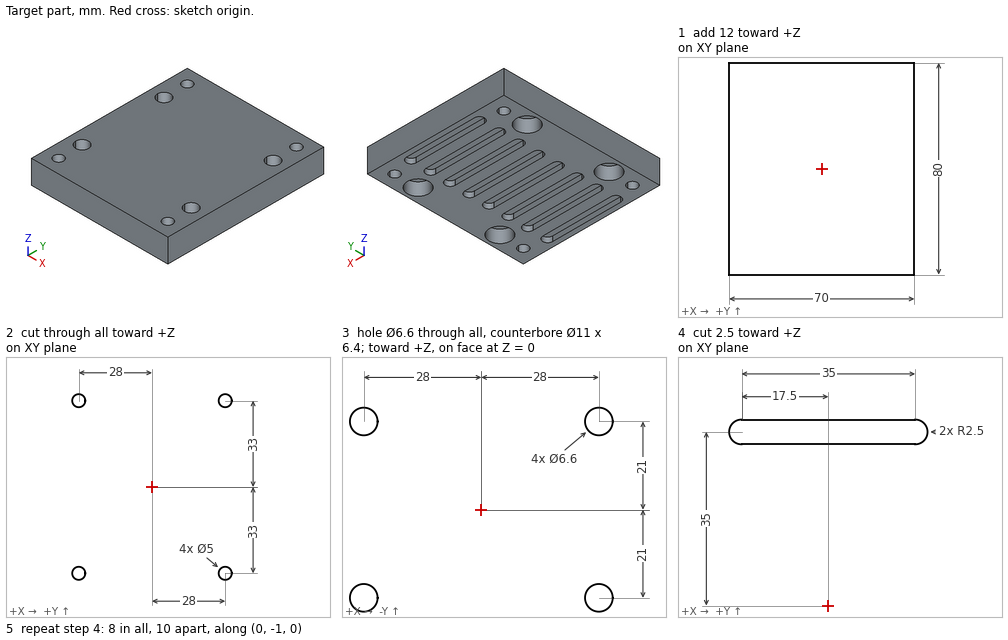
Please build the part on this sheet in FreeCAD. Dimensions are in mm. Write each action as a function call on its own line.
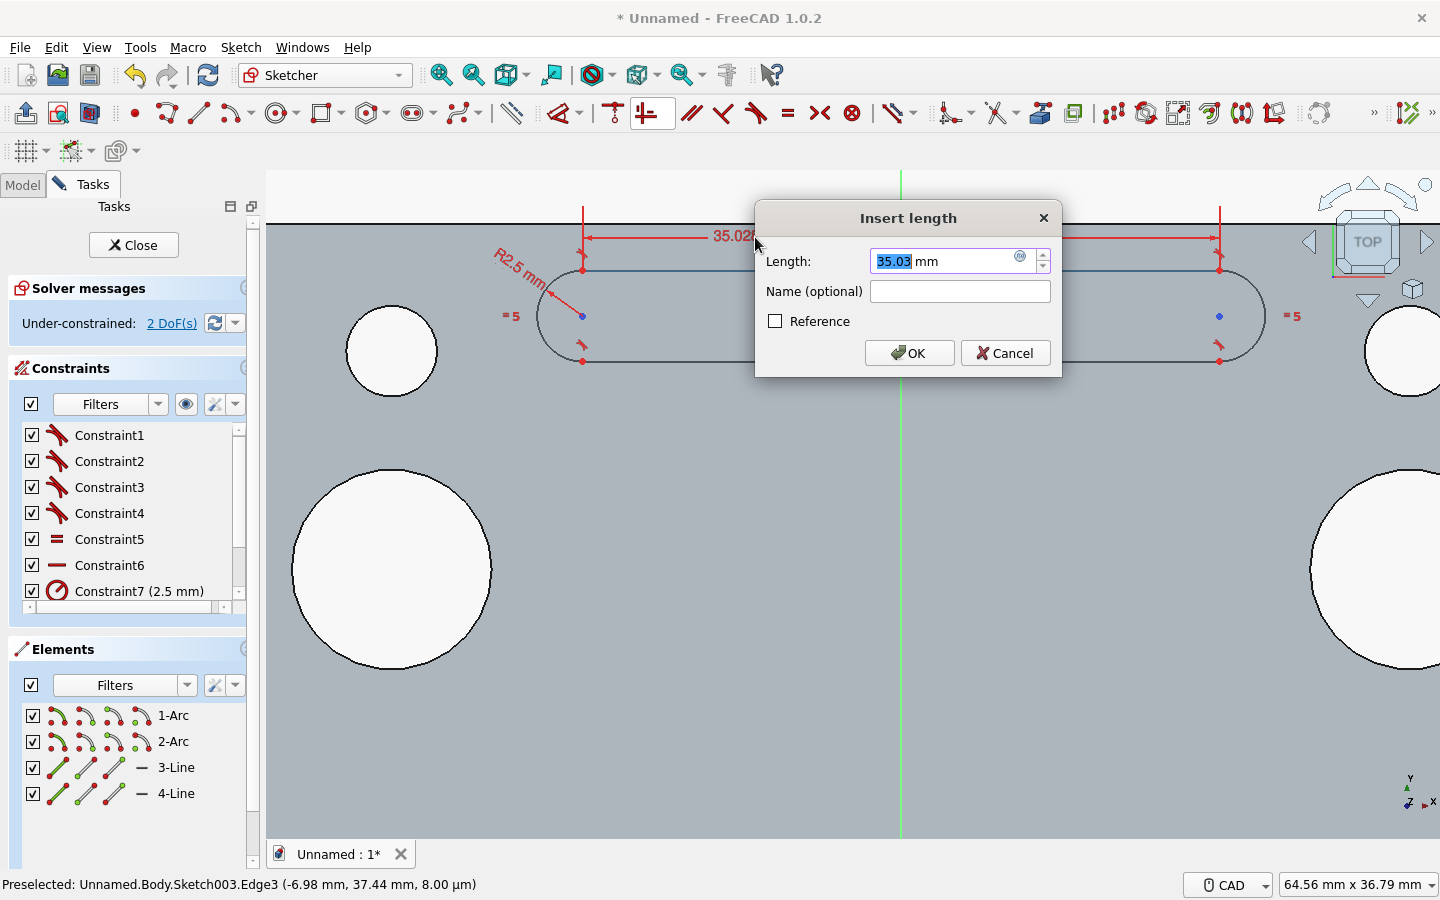
text(35)
key(Return)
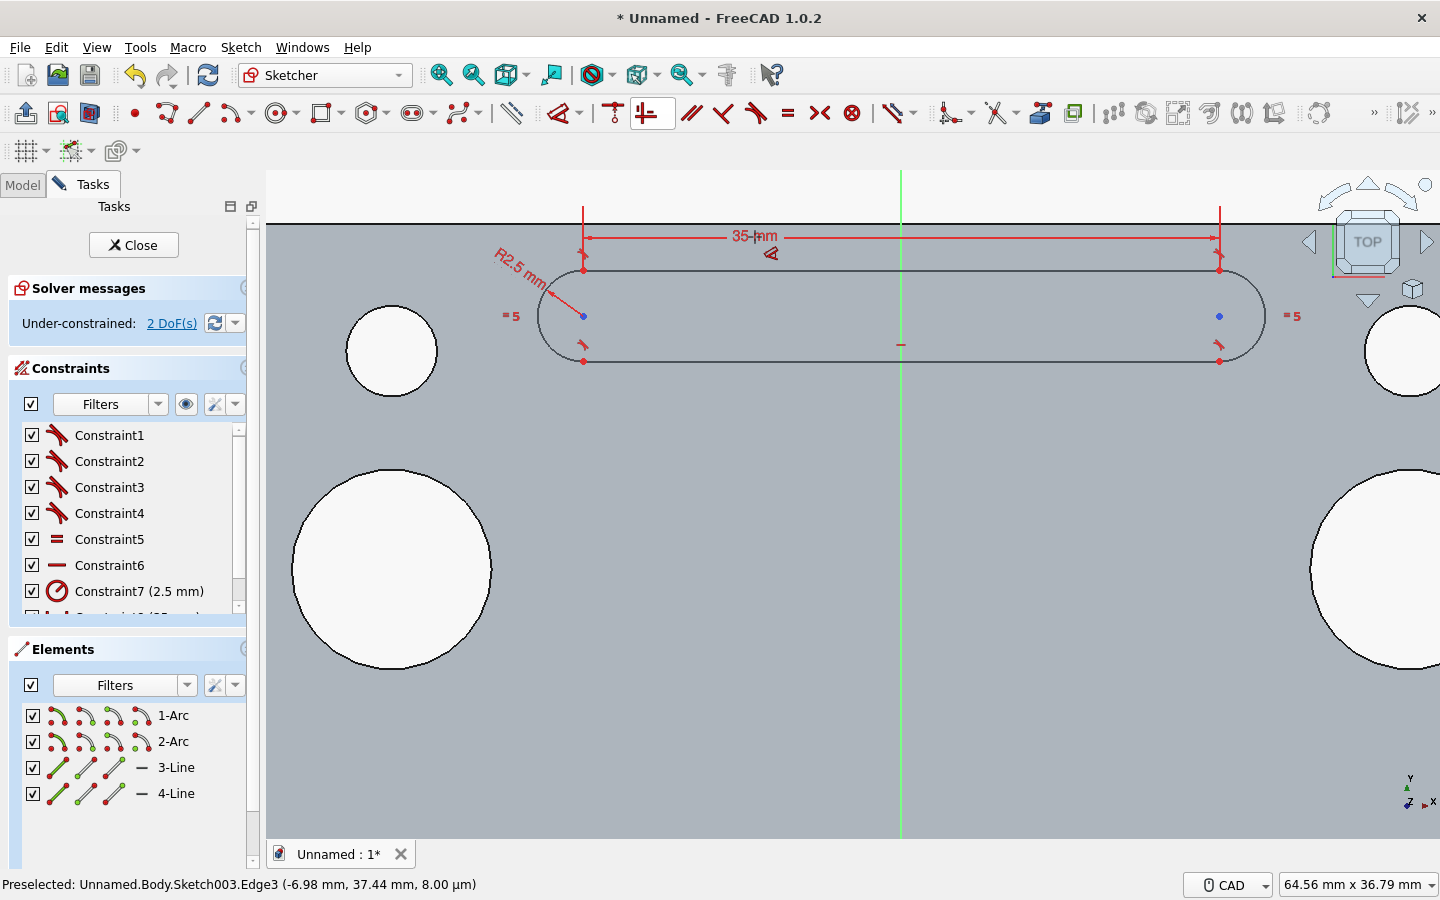
click(583, 316)
click(549, 564)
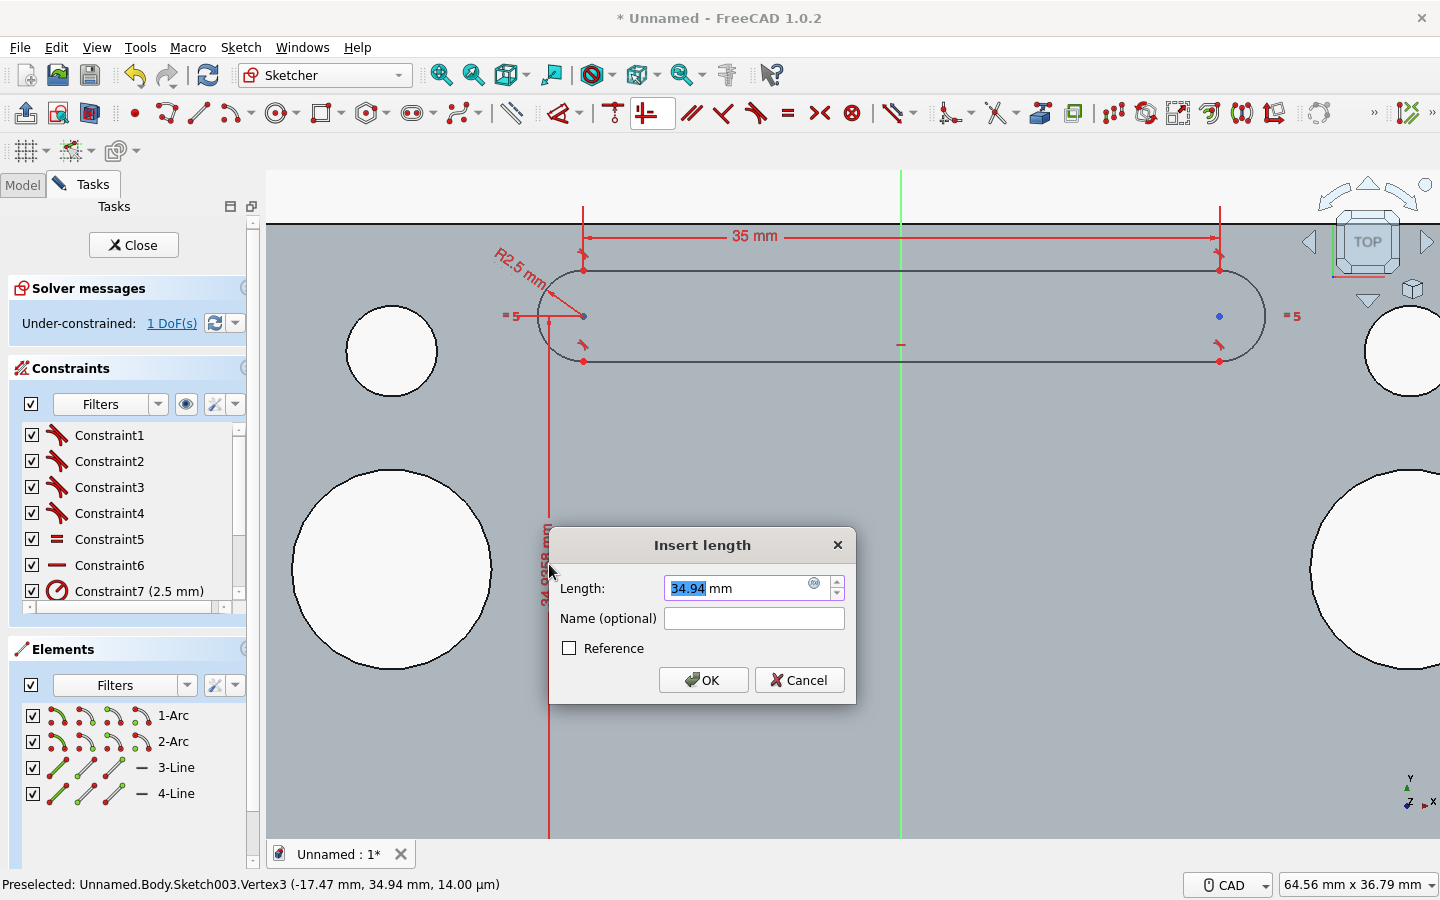
text(35)
key(Return)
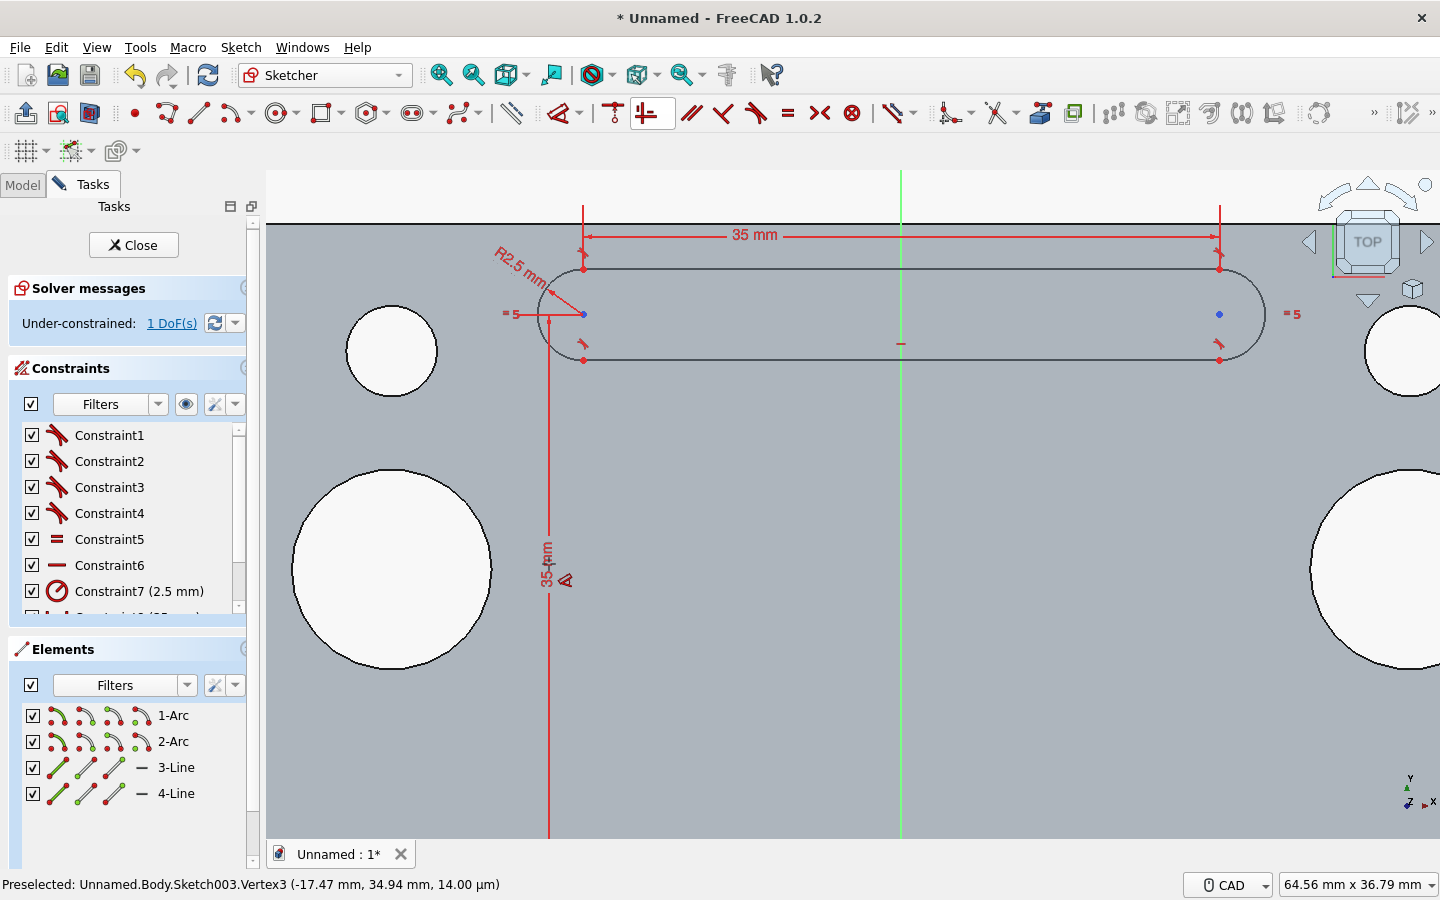
click(583, 269)
click(669, 235)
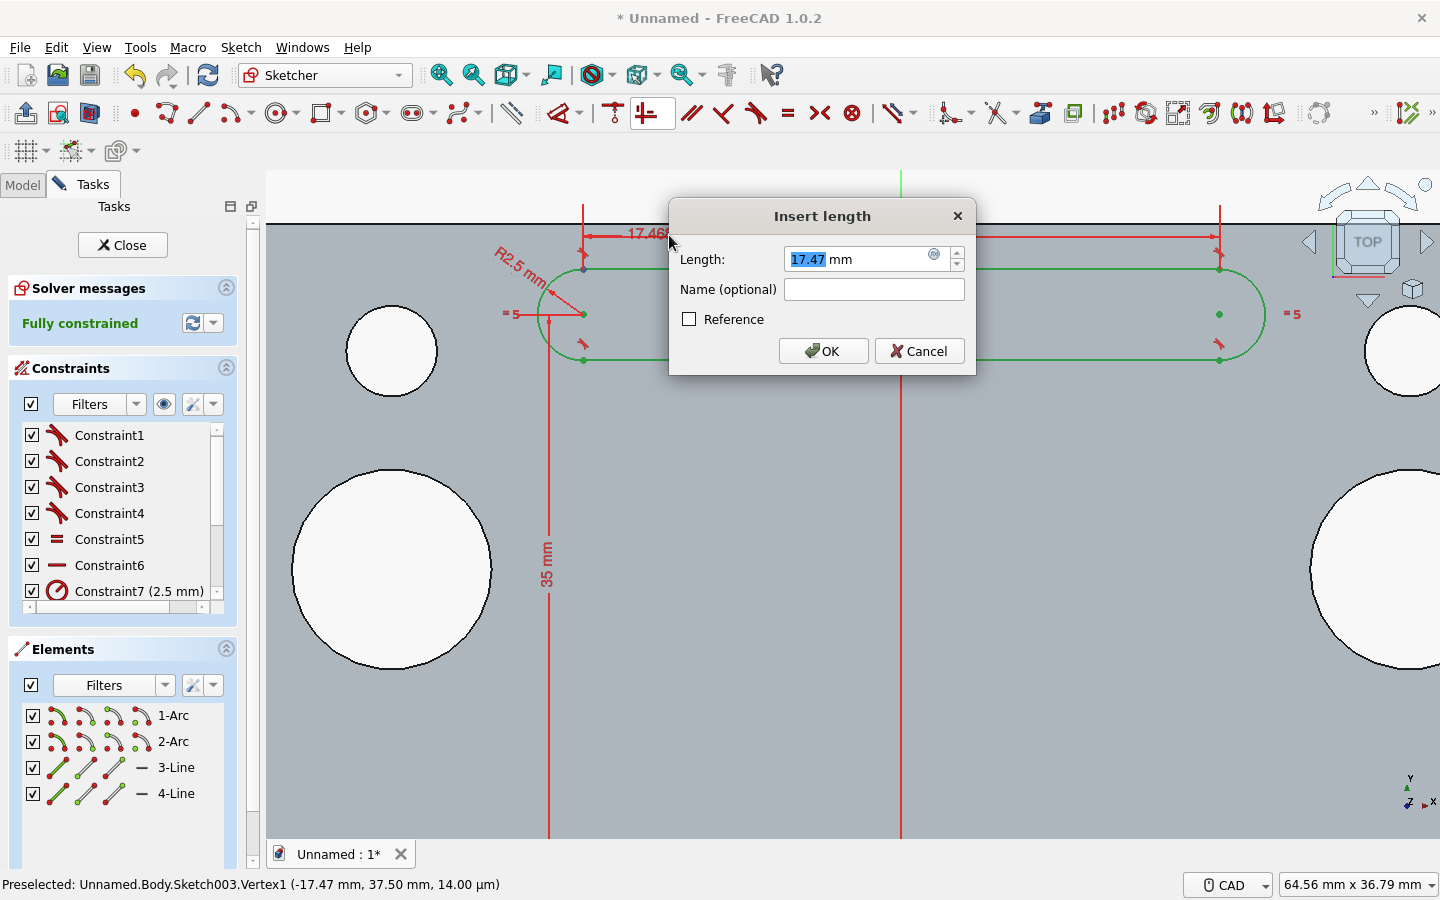
text(17.5)
key(Return)
key(Escape)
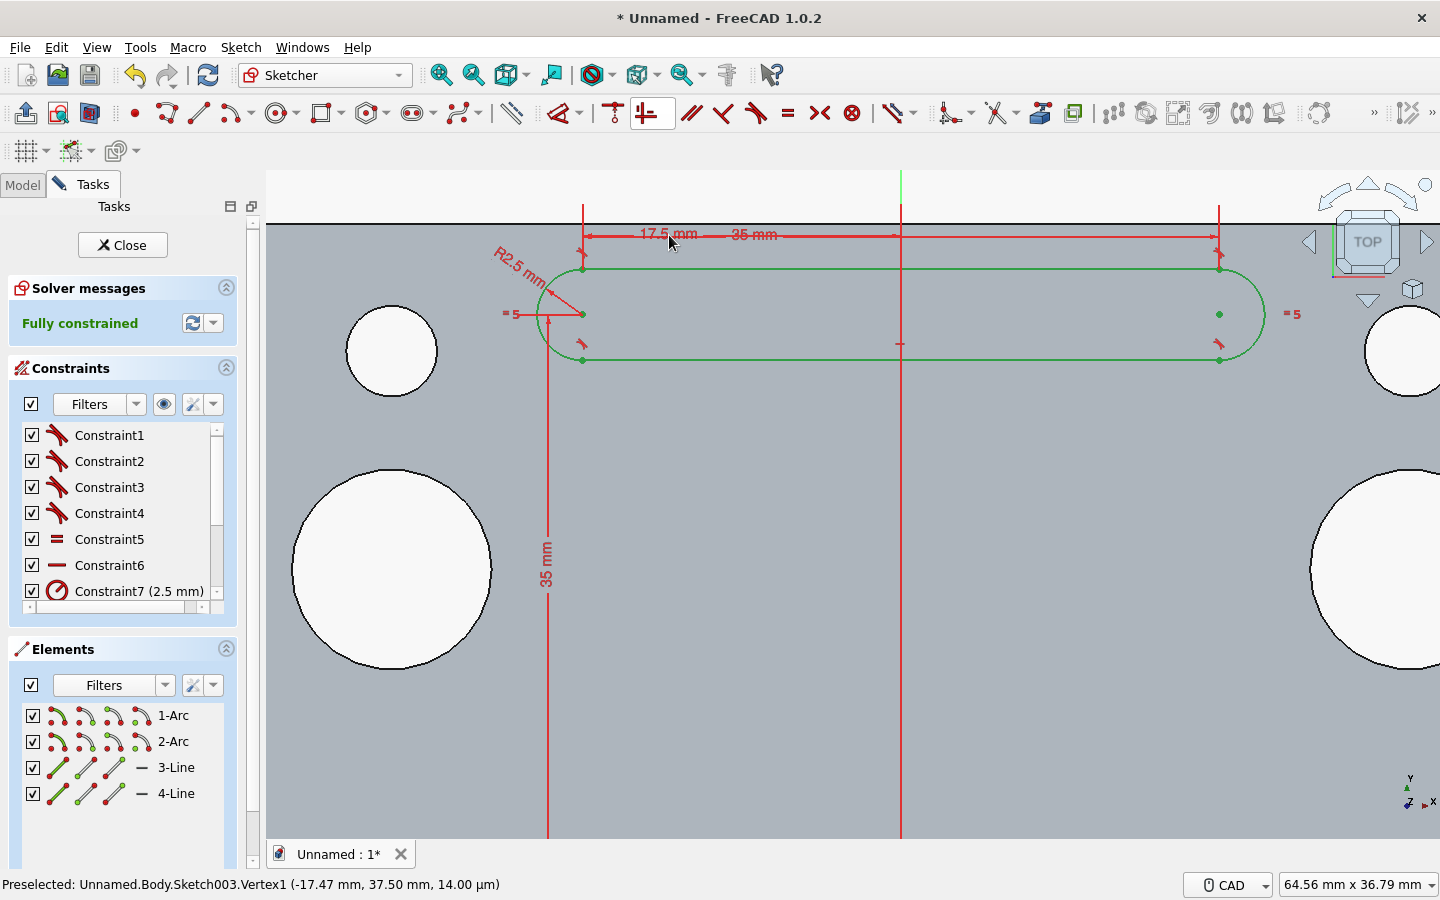
click(123, 245)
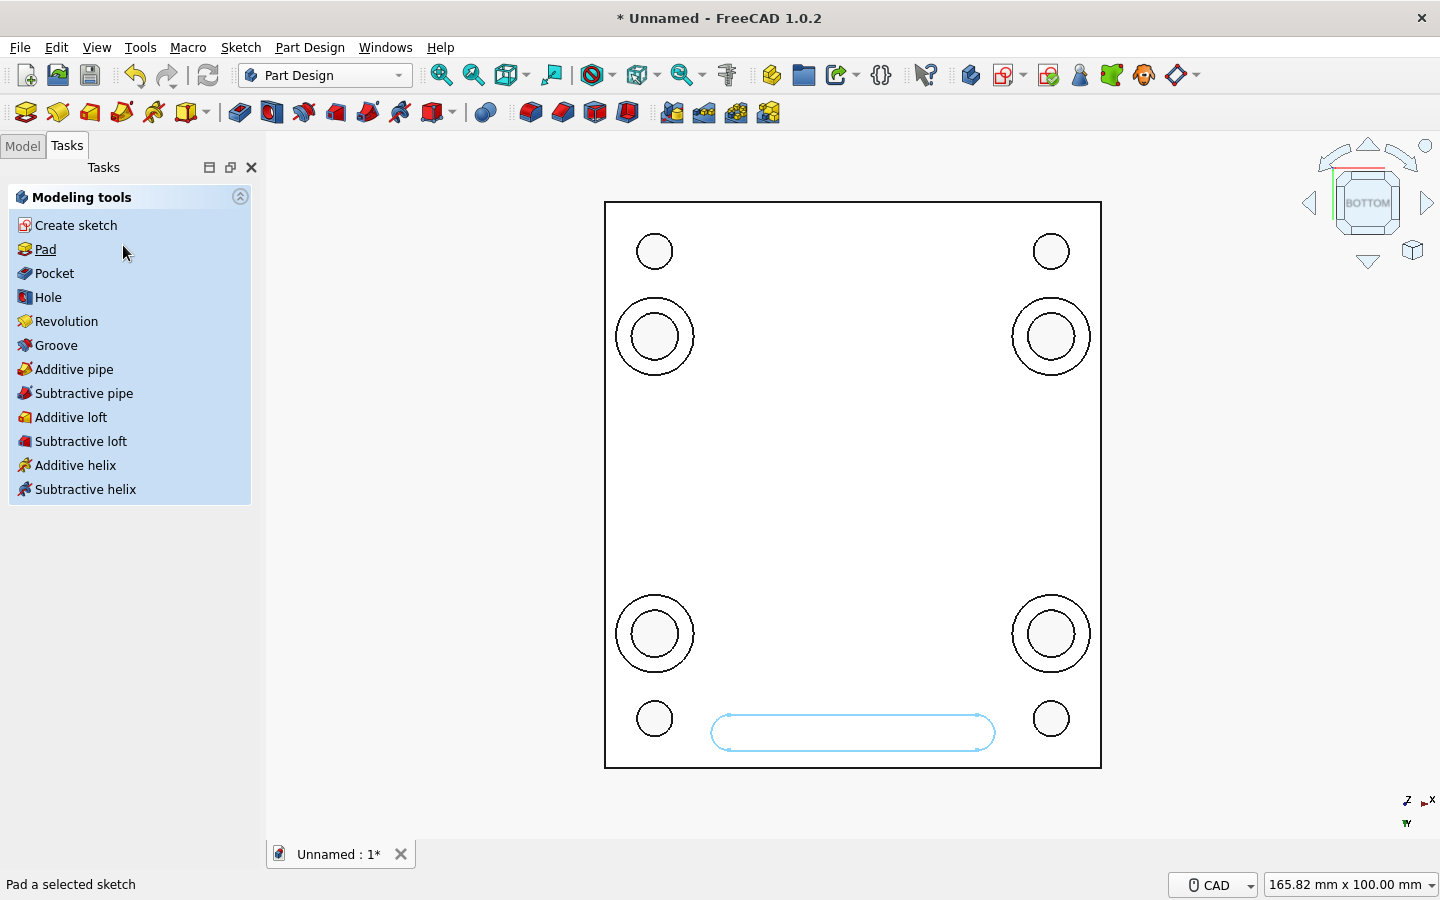
click(240, 112)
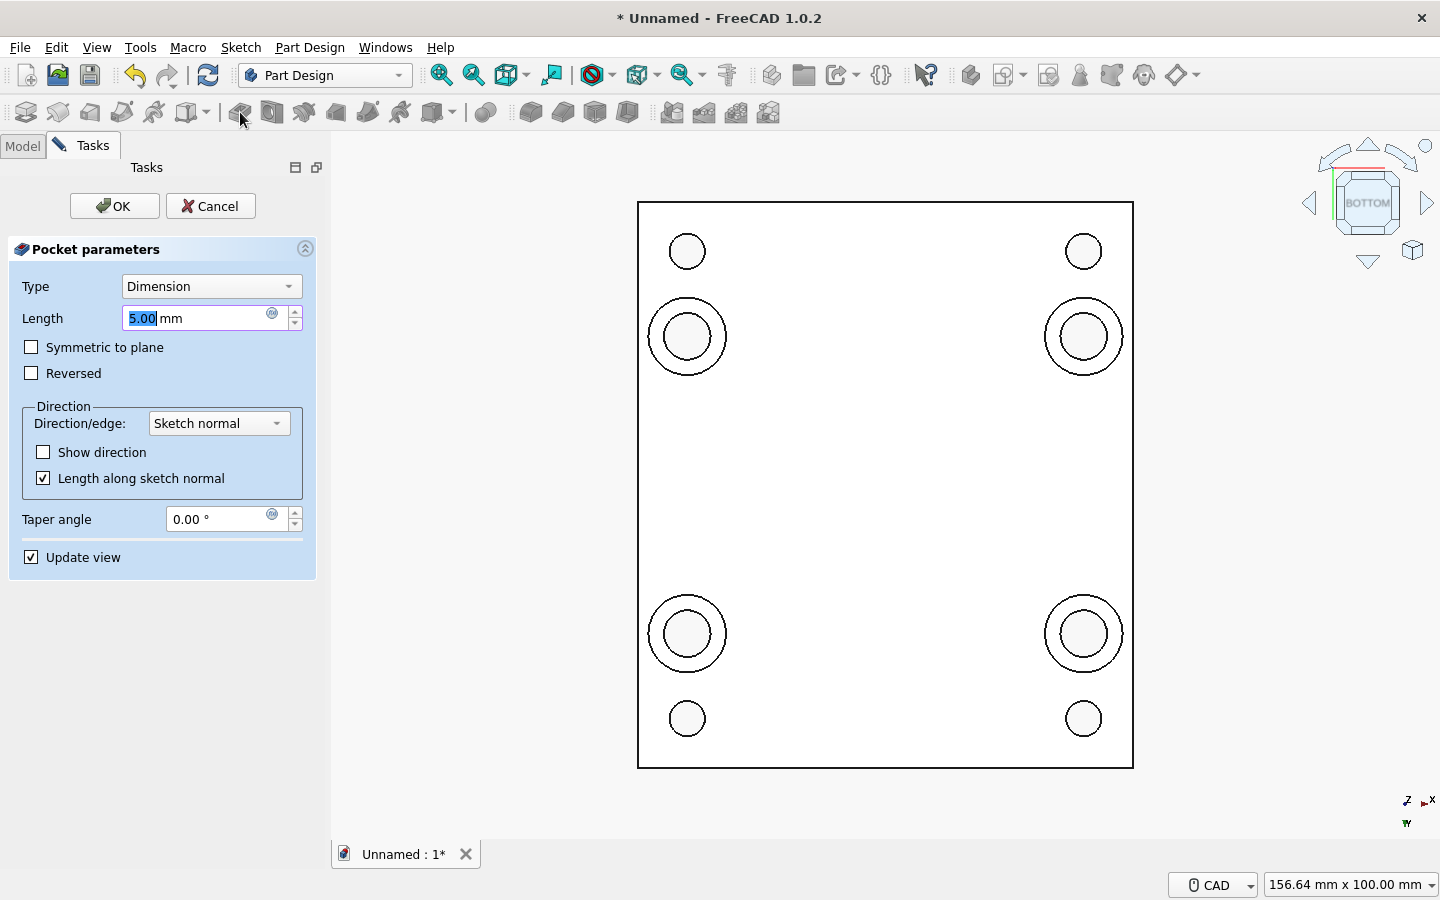
text(2.5)
key(Tab)